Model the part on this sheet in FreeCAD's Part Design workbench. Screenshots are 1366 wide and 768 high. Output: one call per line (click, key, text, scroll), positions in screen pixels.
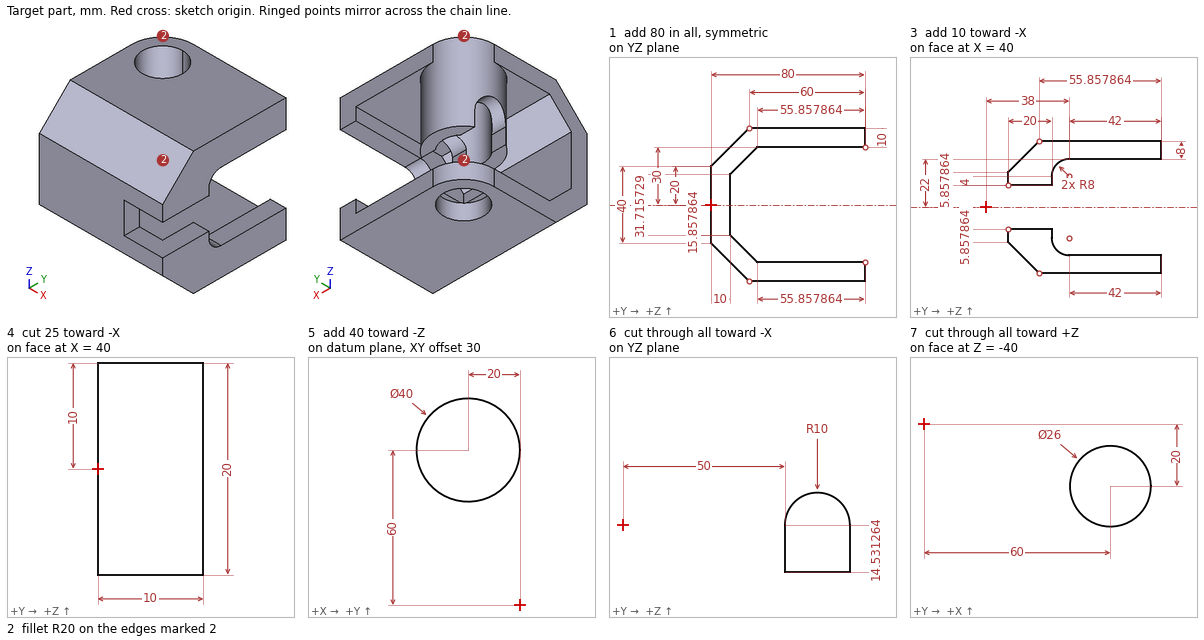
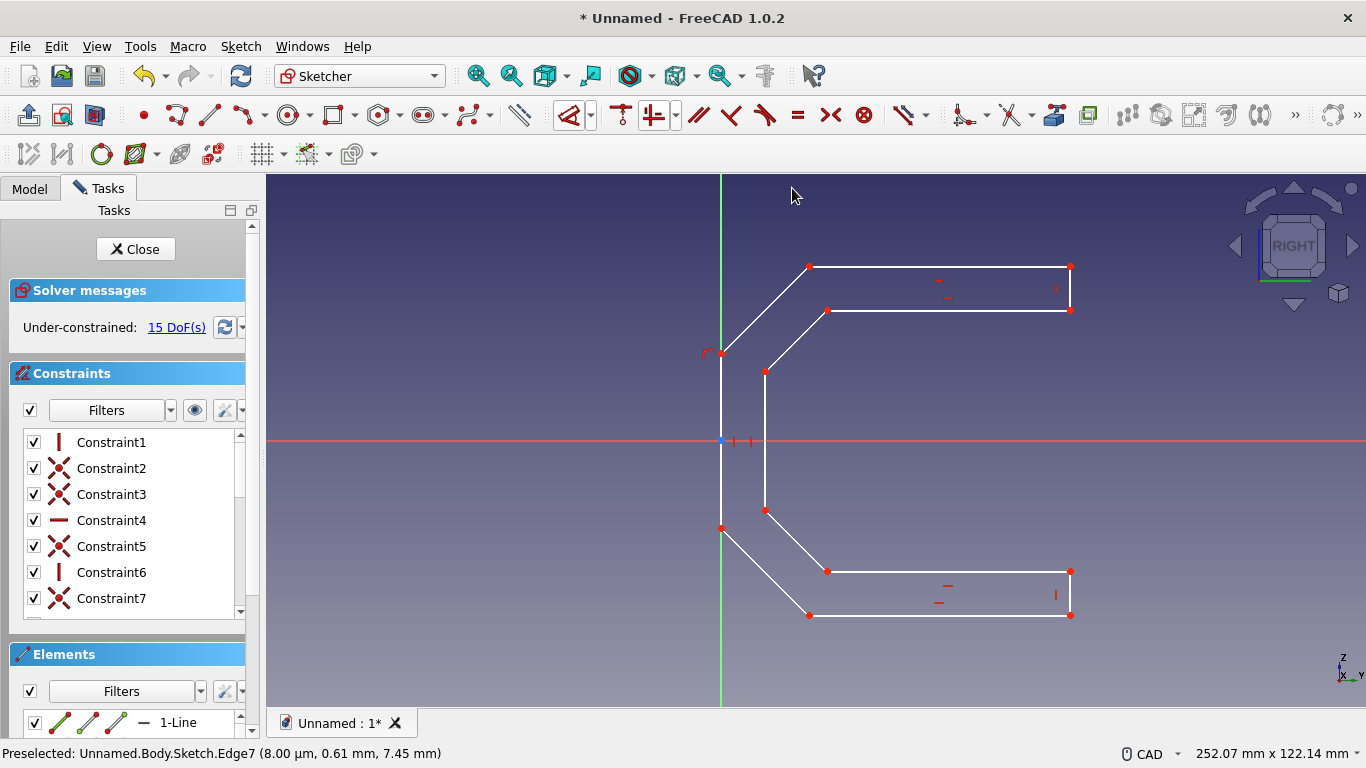
click(809, 267)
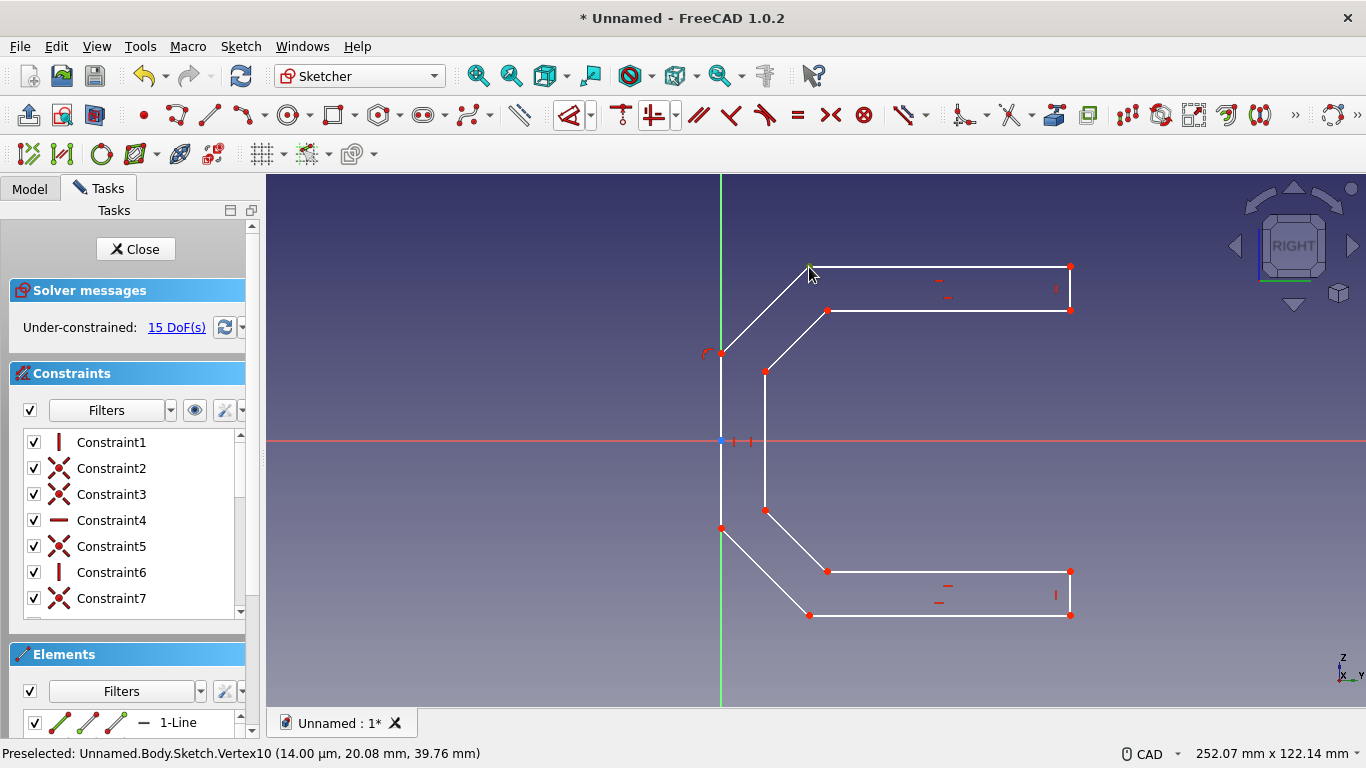
click(809, 616)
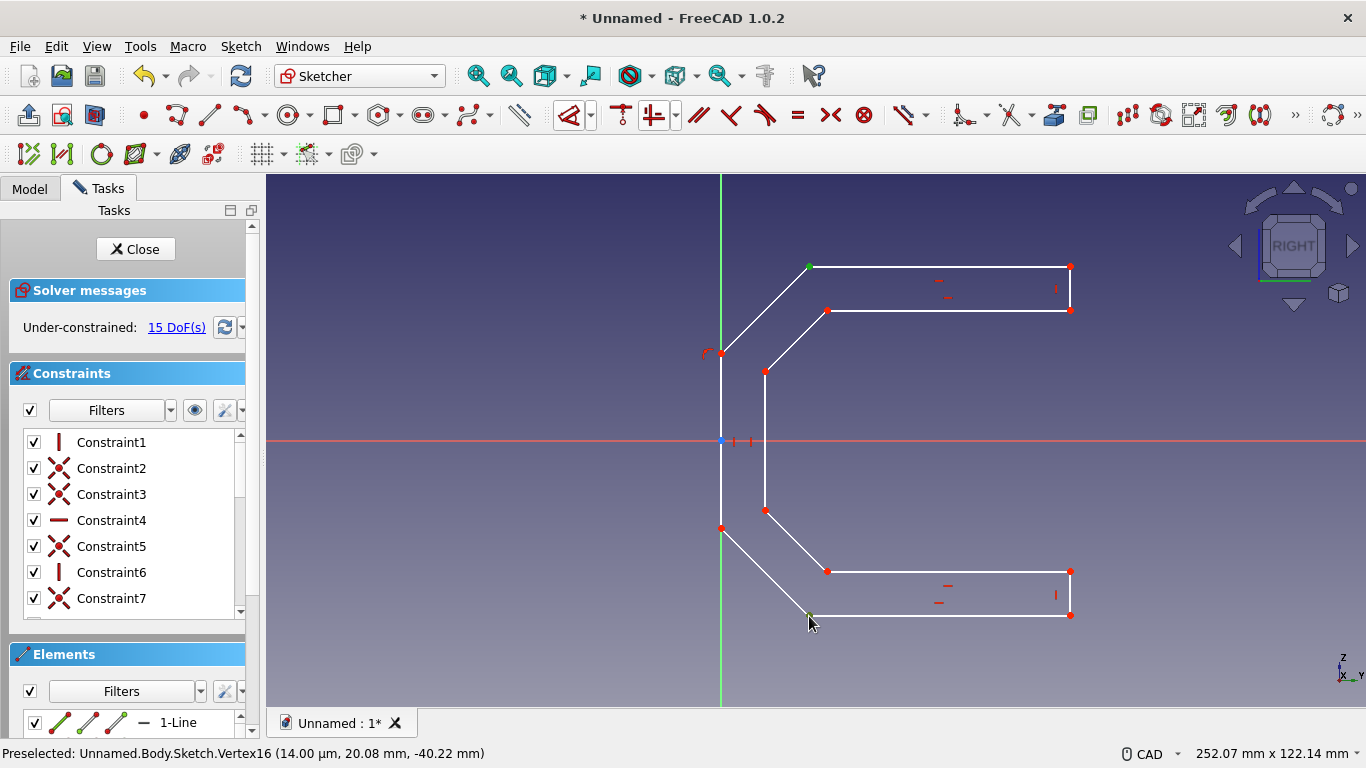
click(359, 440)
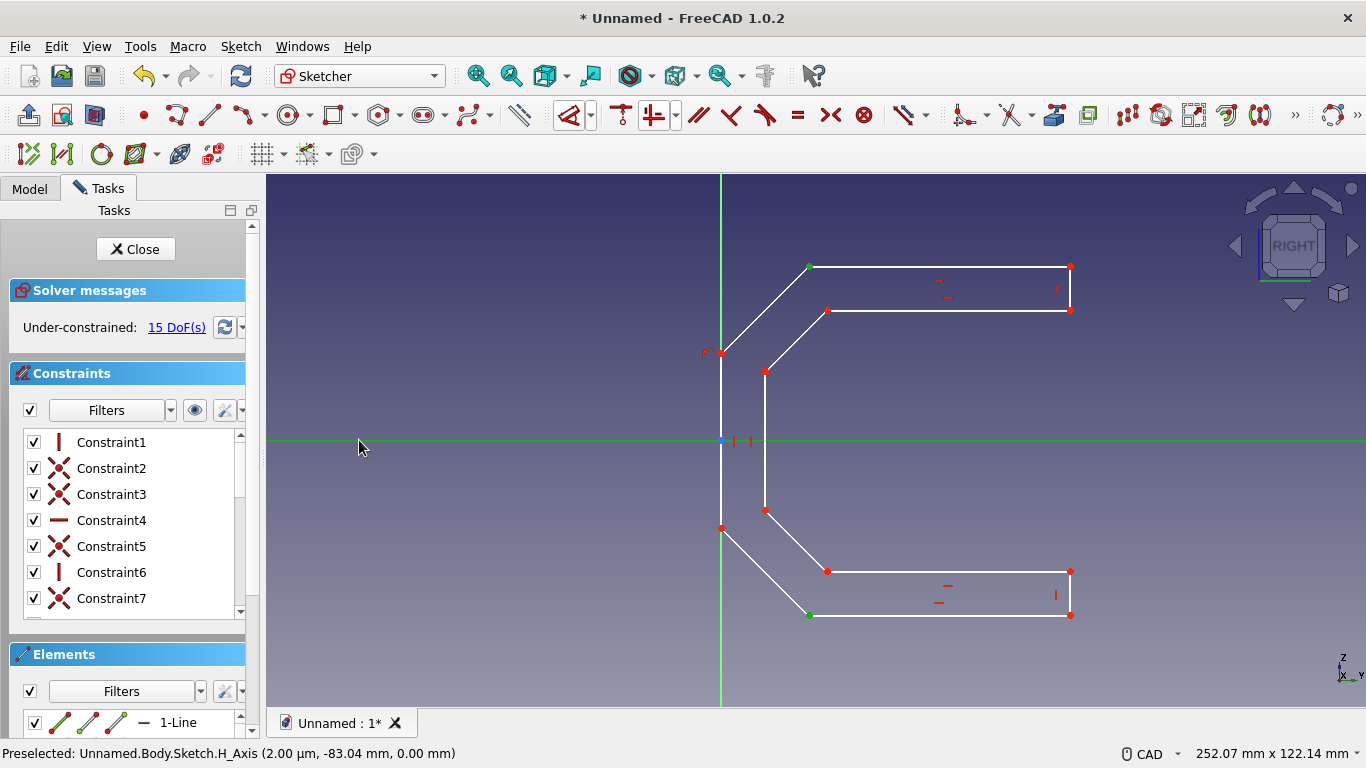
click(831, 116)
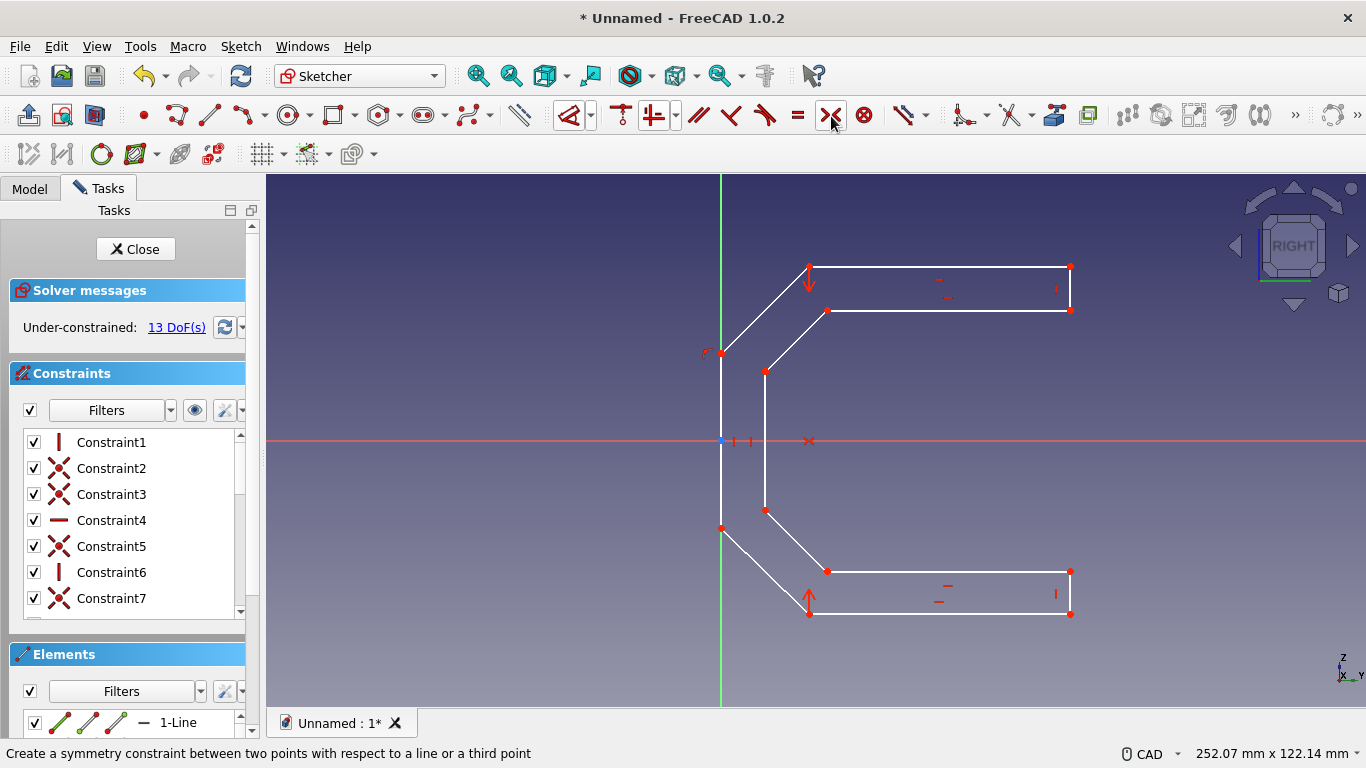
click(1070, 311)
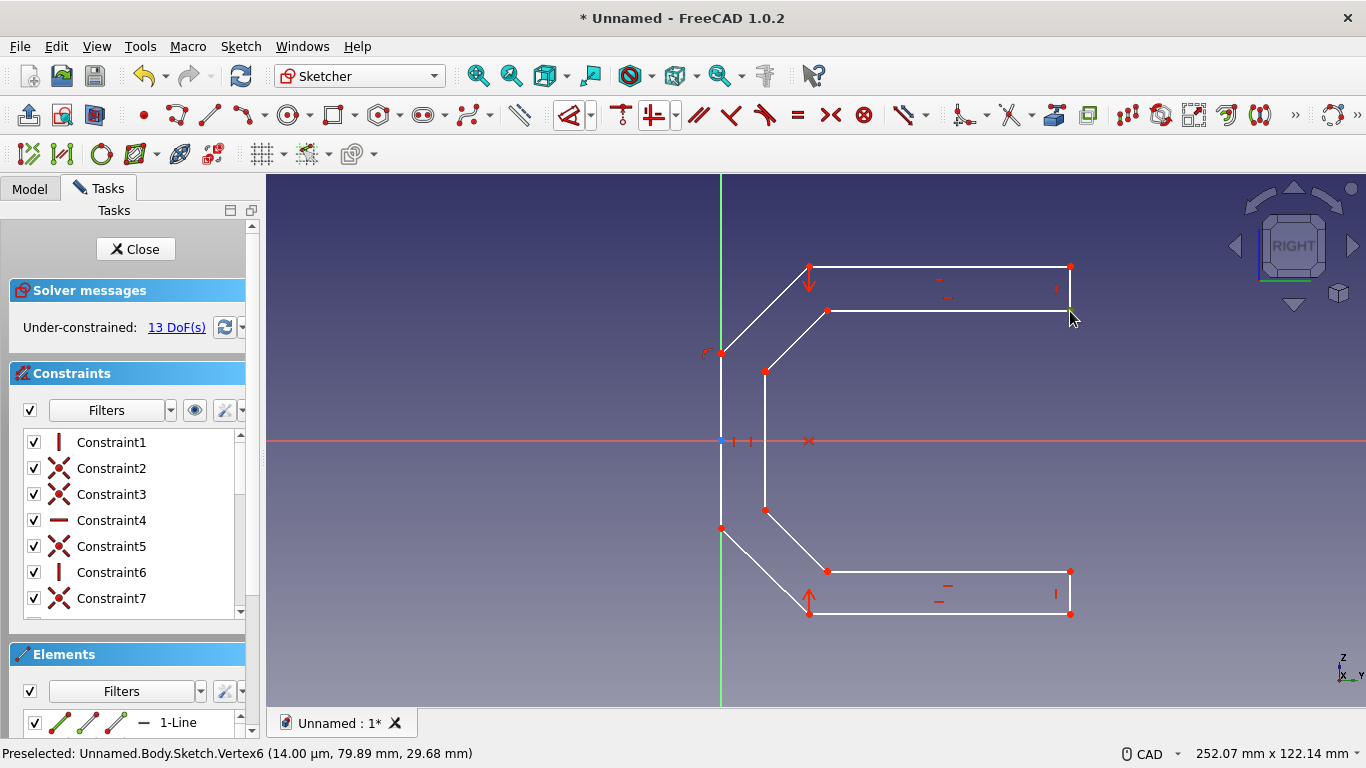
click(1070, 572)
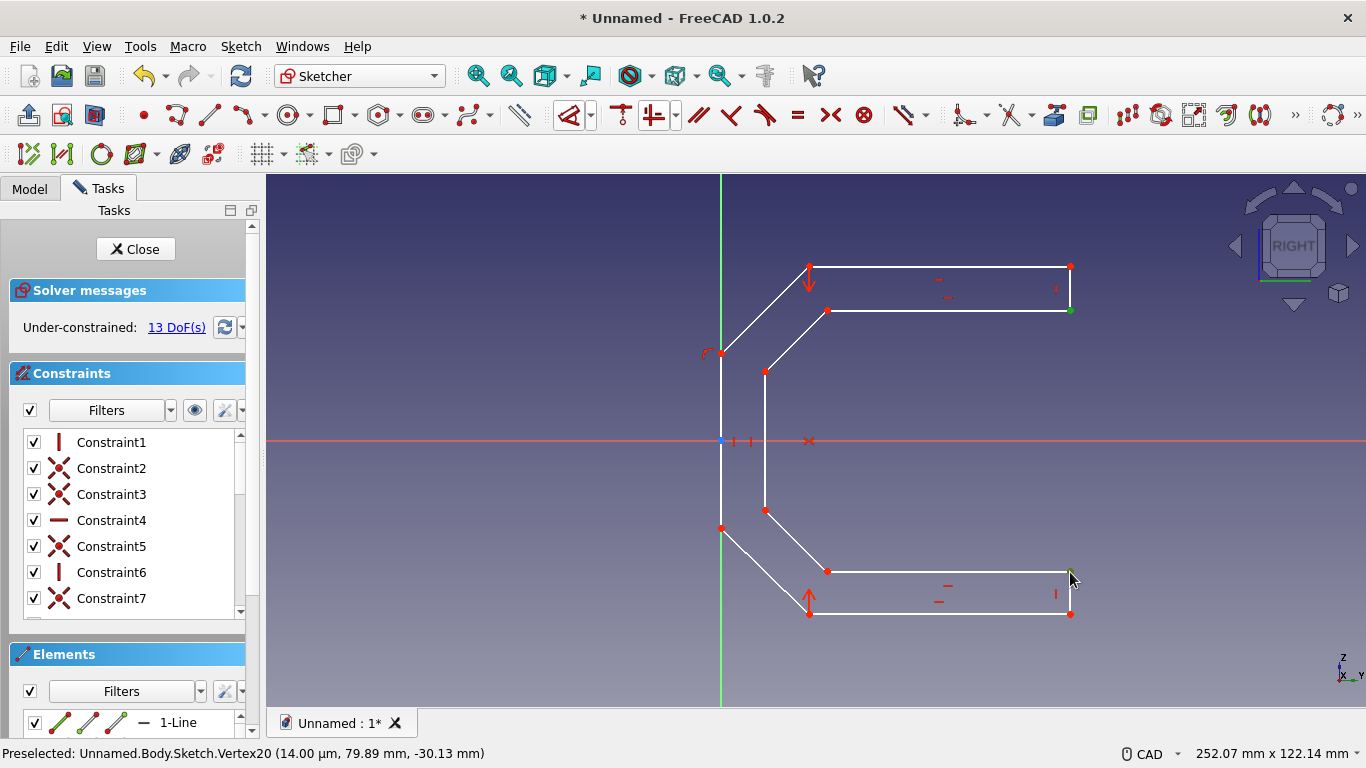
click(359, 440)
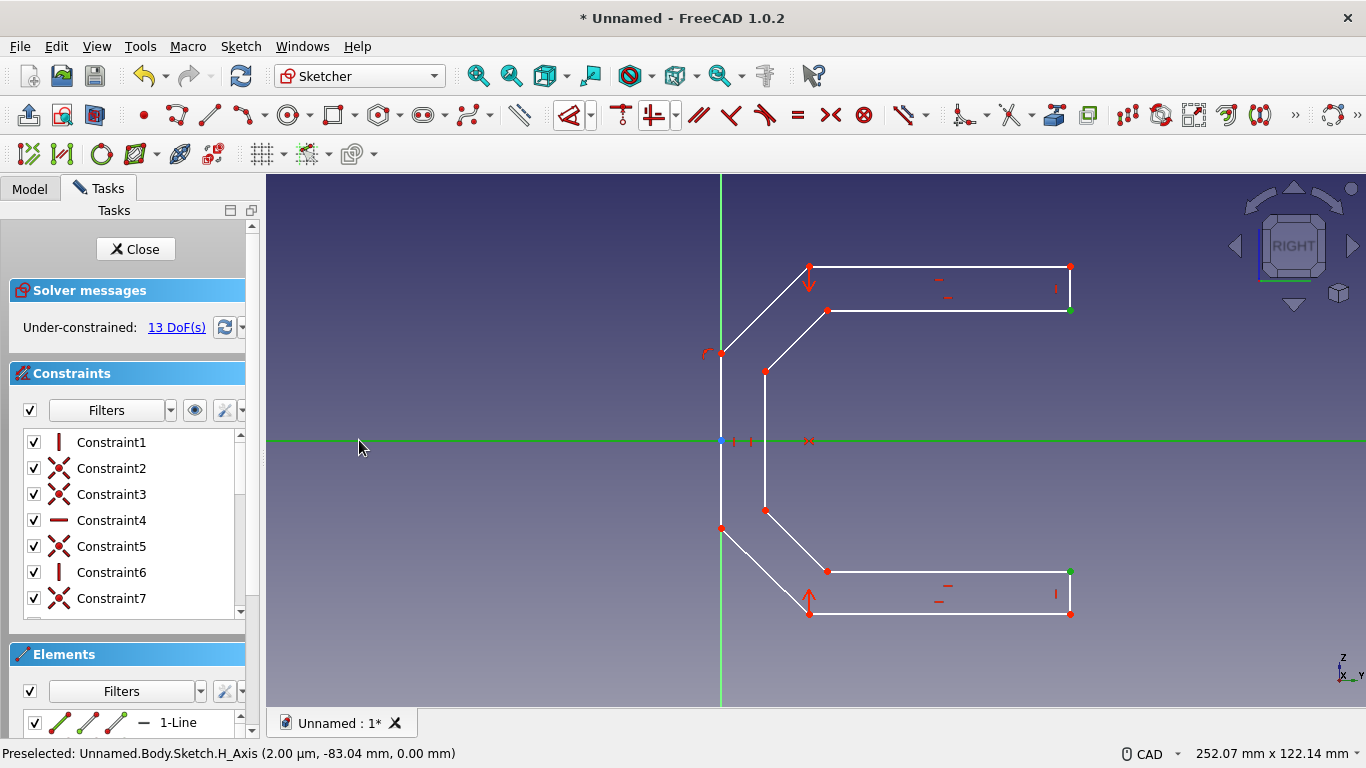
click(831, 116)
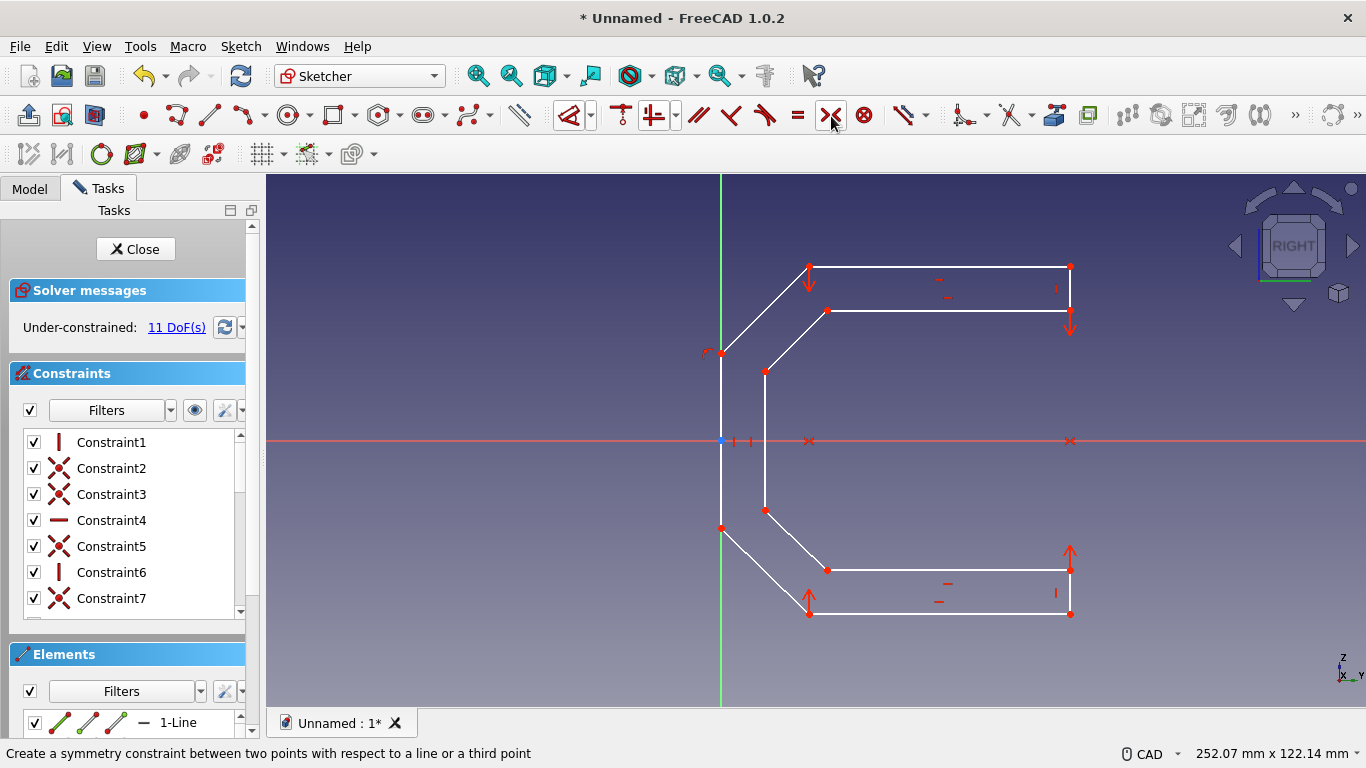
click(1070, 297)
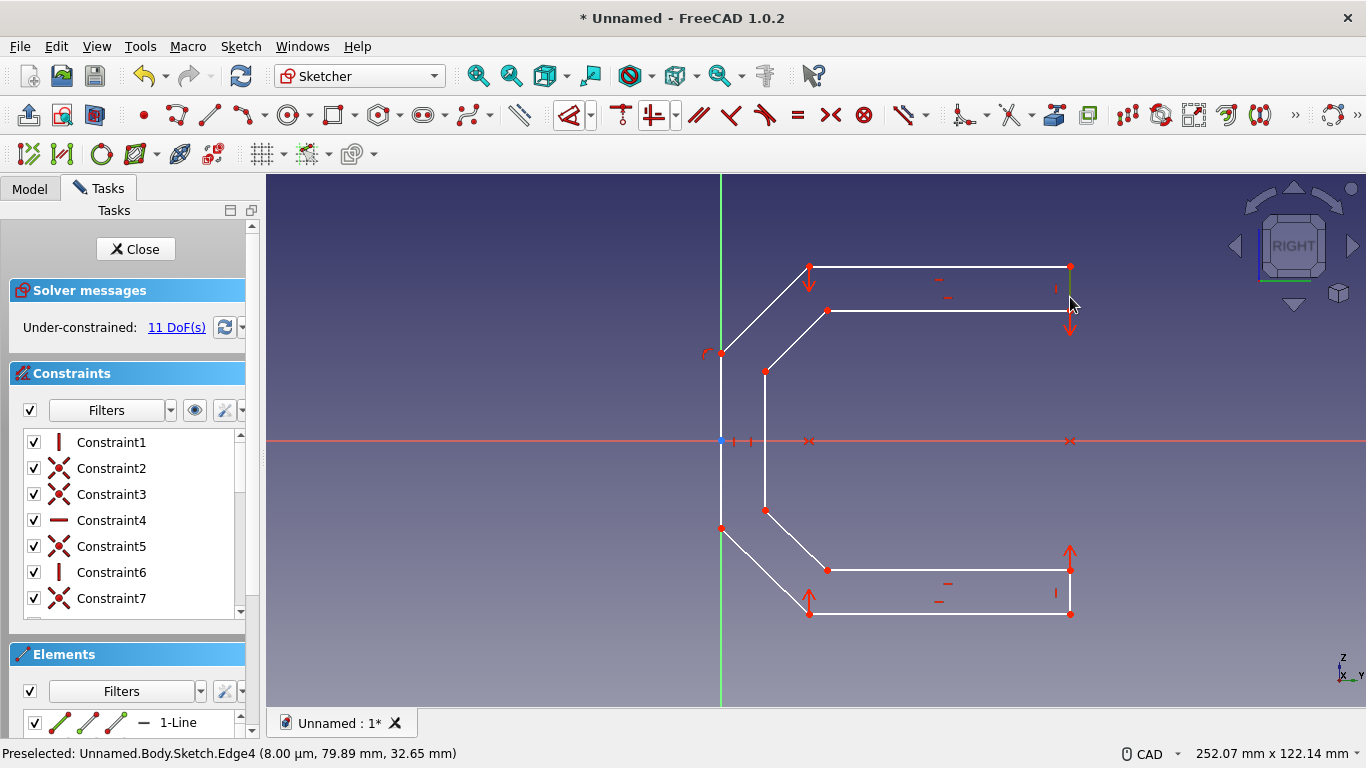
click(590, 116)